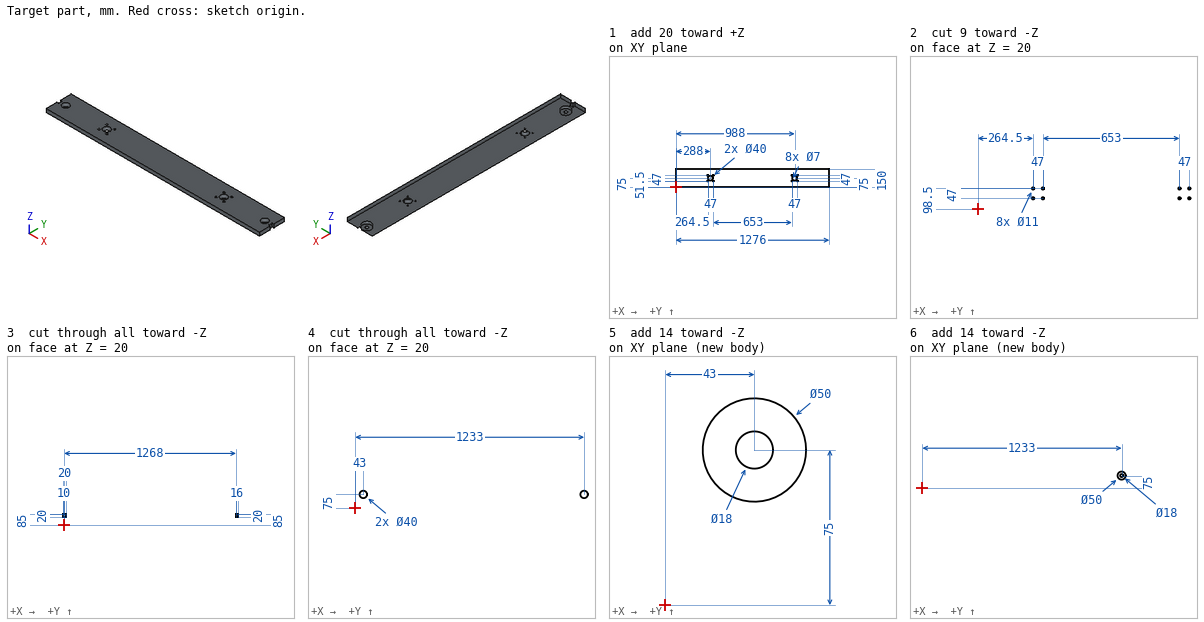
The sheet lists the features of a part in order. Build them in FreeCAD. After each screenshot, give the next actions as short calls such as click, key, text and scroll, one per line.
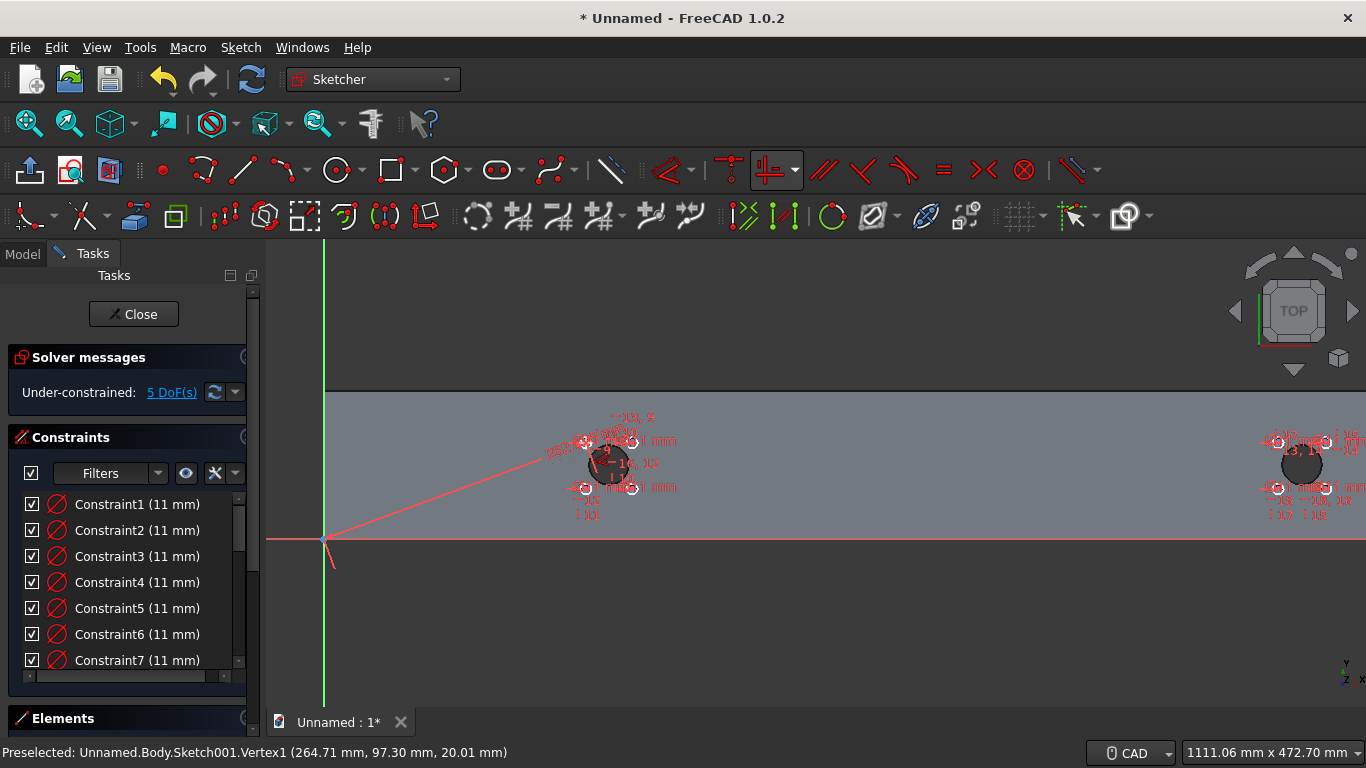
click(632, 443)
click(609, 409)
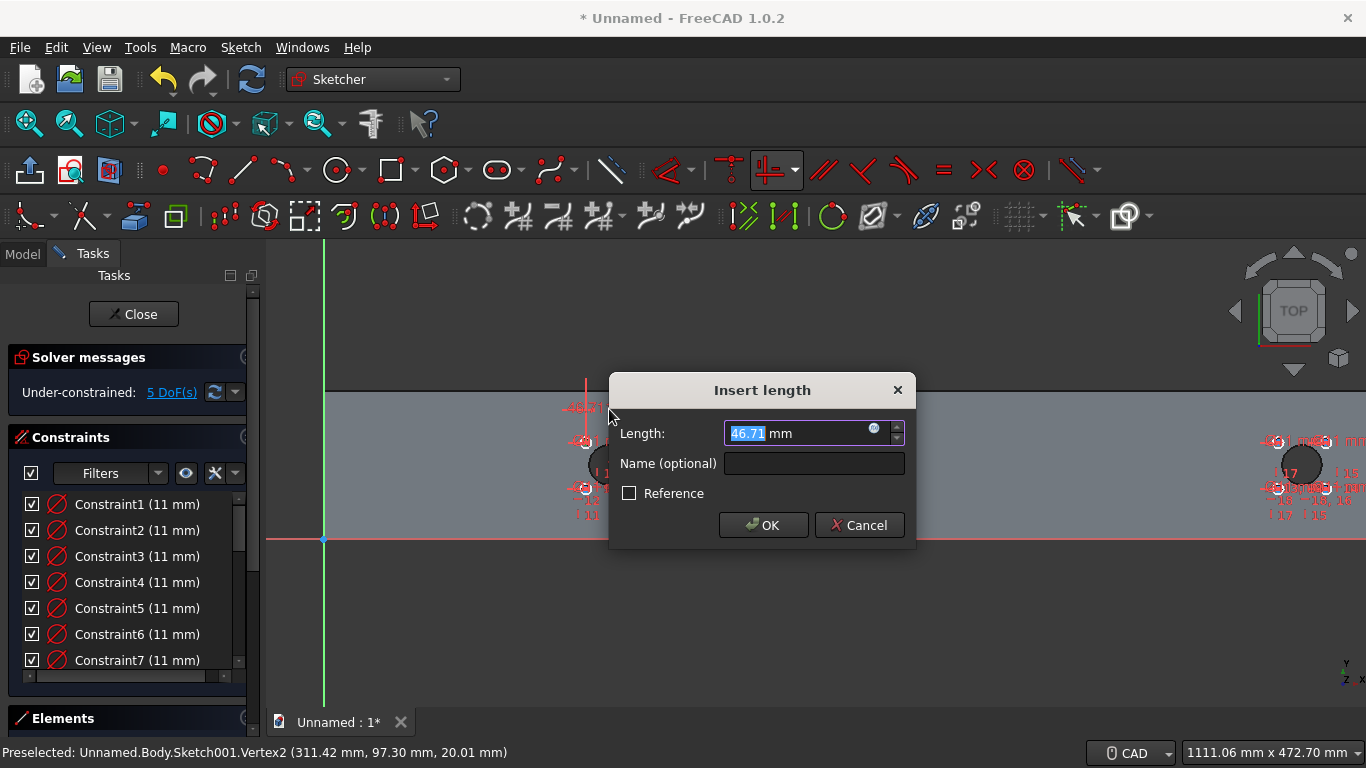
text(47)
key(Return)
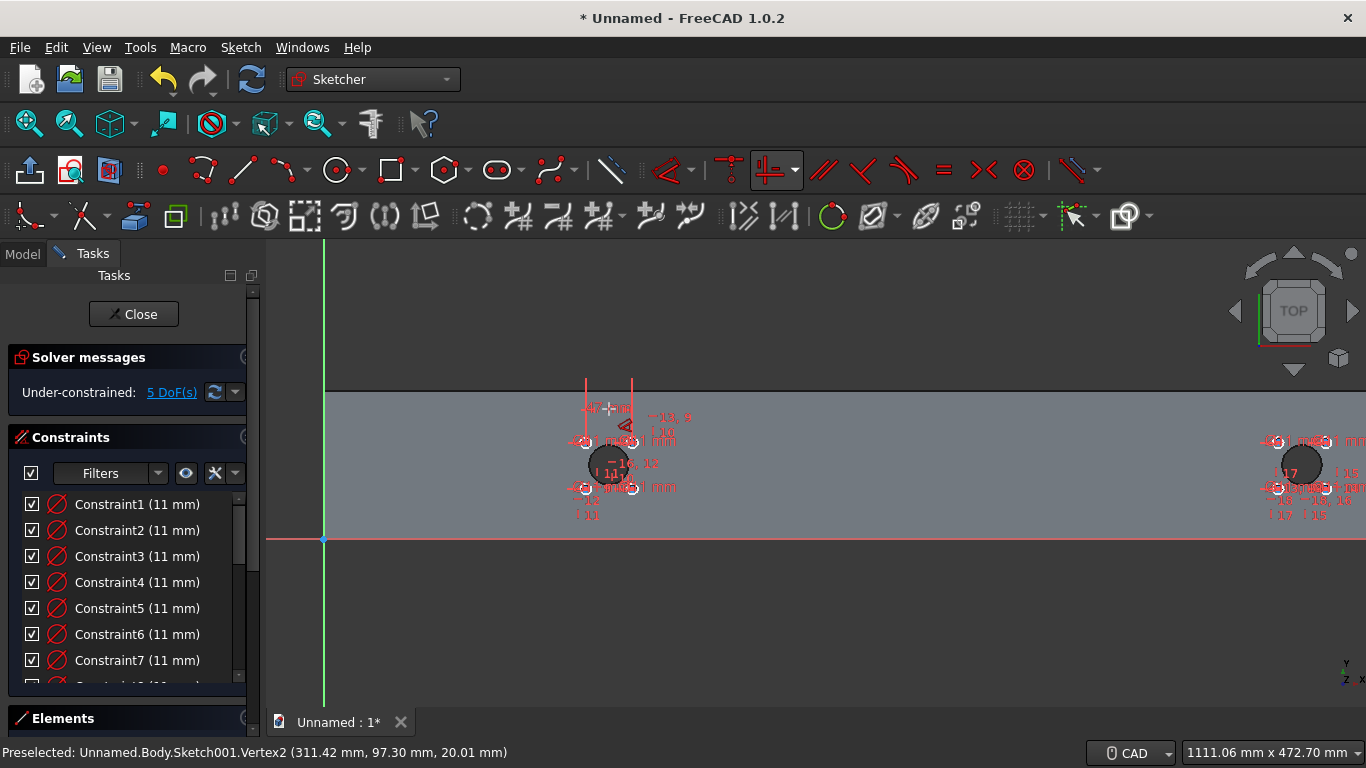
click(632, 443)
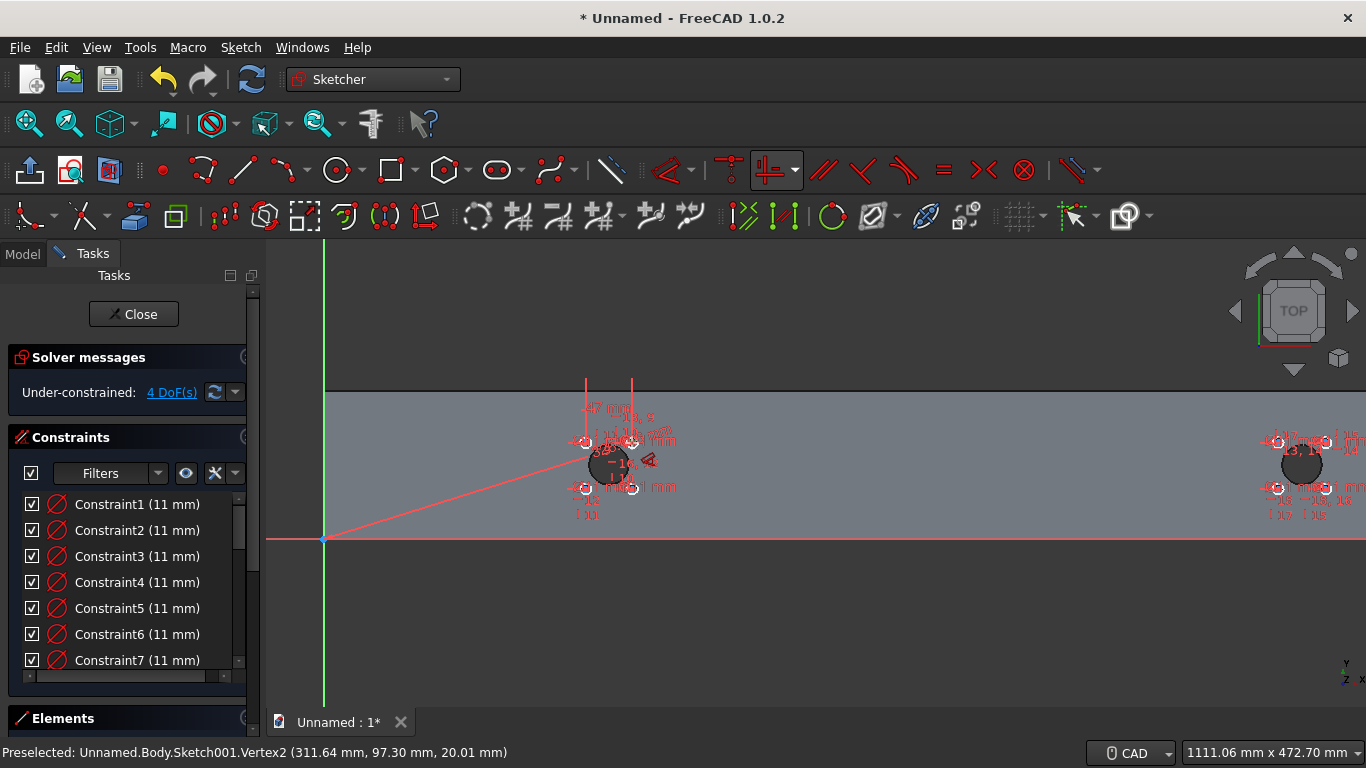
click(632, 489)
click(598, 466)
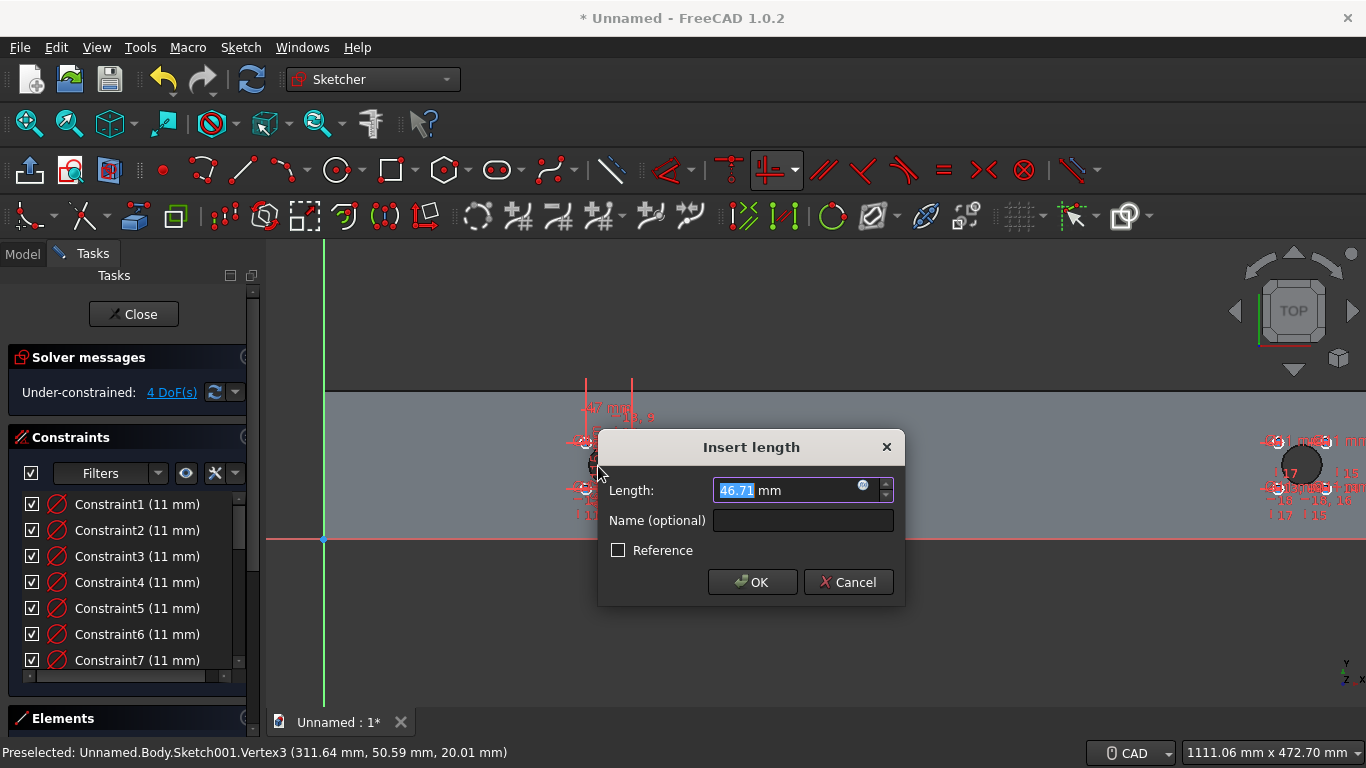
text(47)
key(Return)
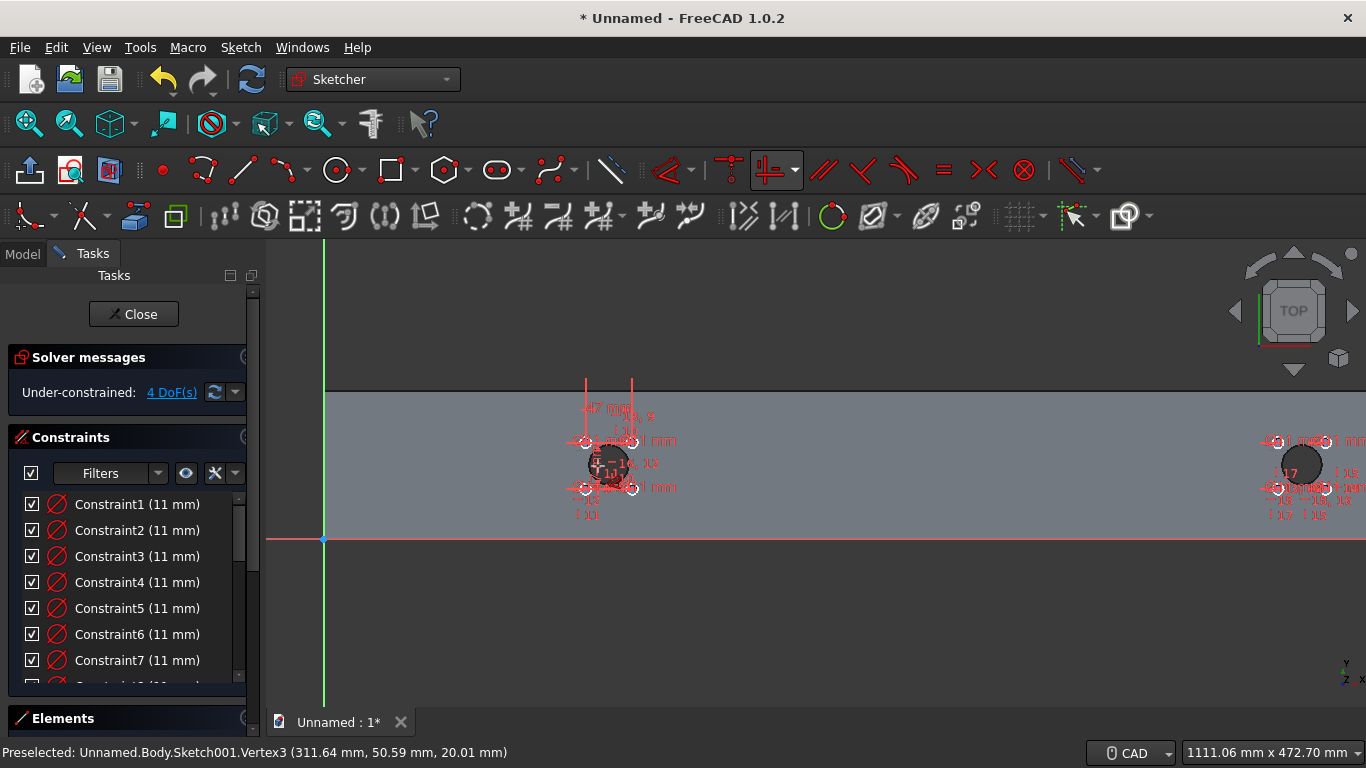
scroll(585, 443, down, 2)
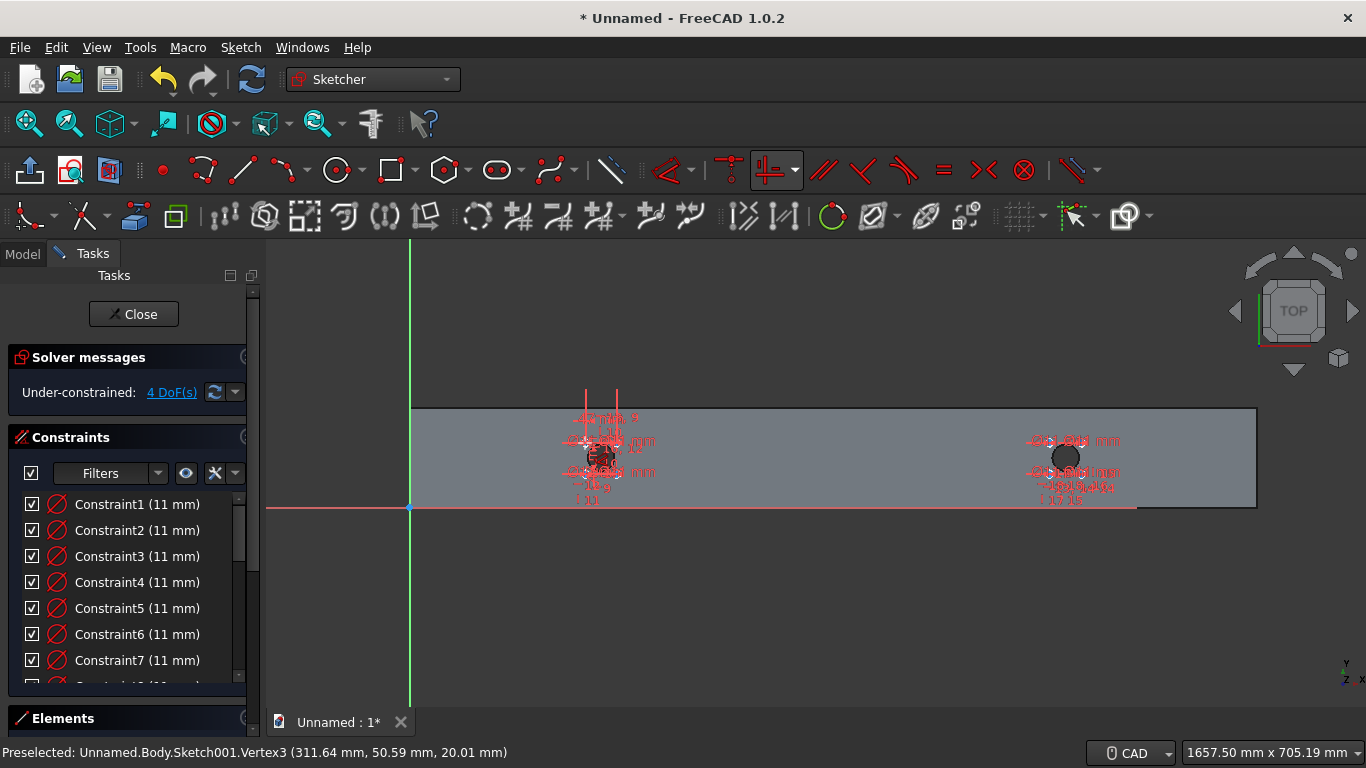
scroll(1050, 443, up, 2)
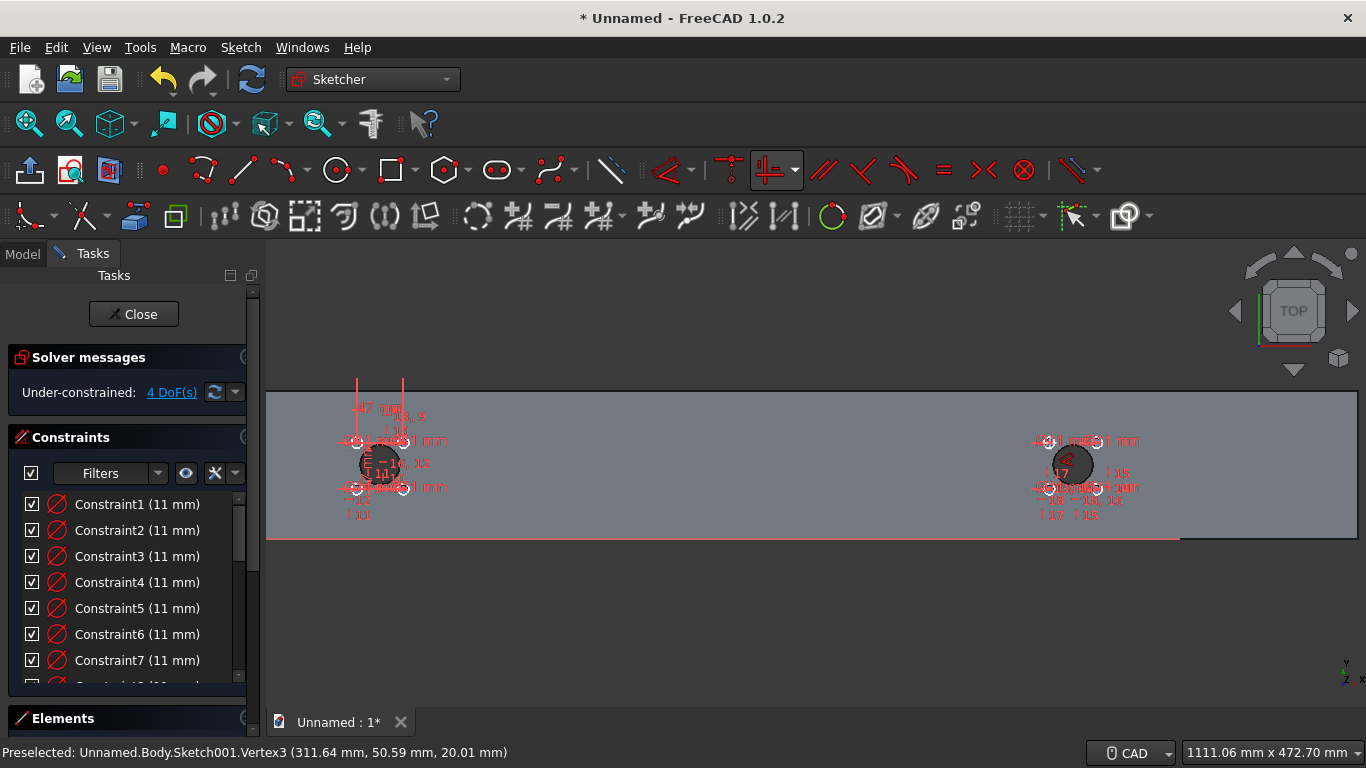
click(1049, 443)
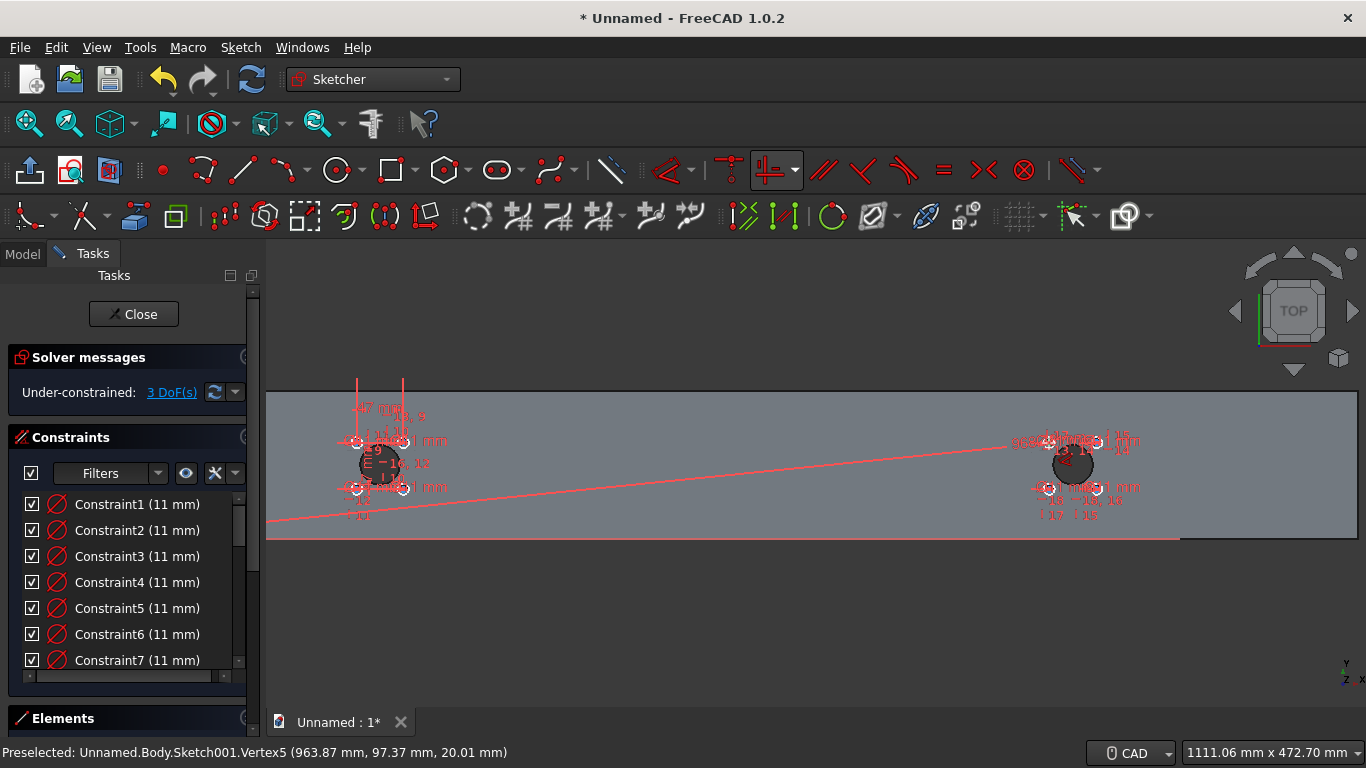
click(1097, 443)
click(1073, 409)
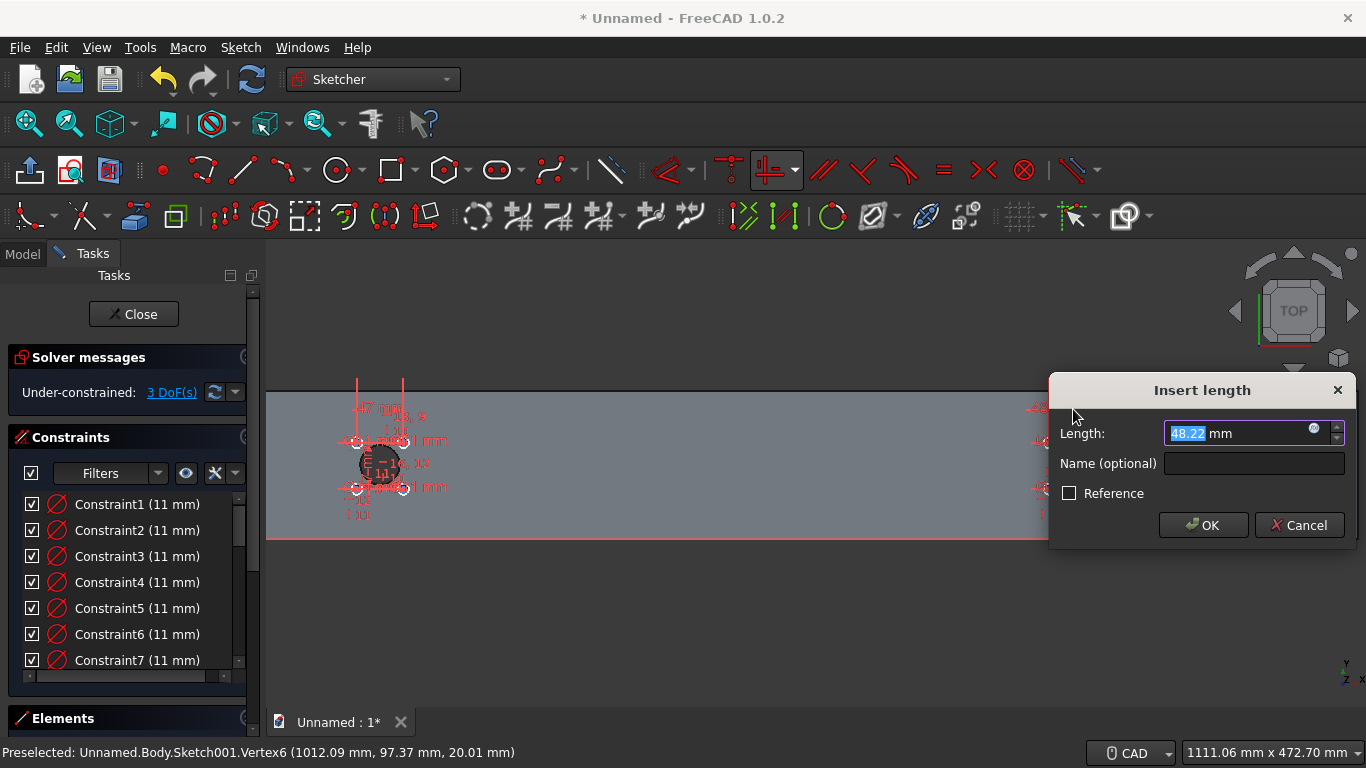
text(47)
key(Return)